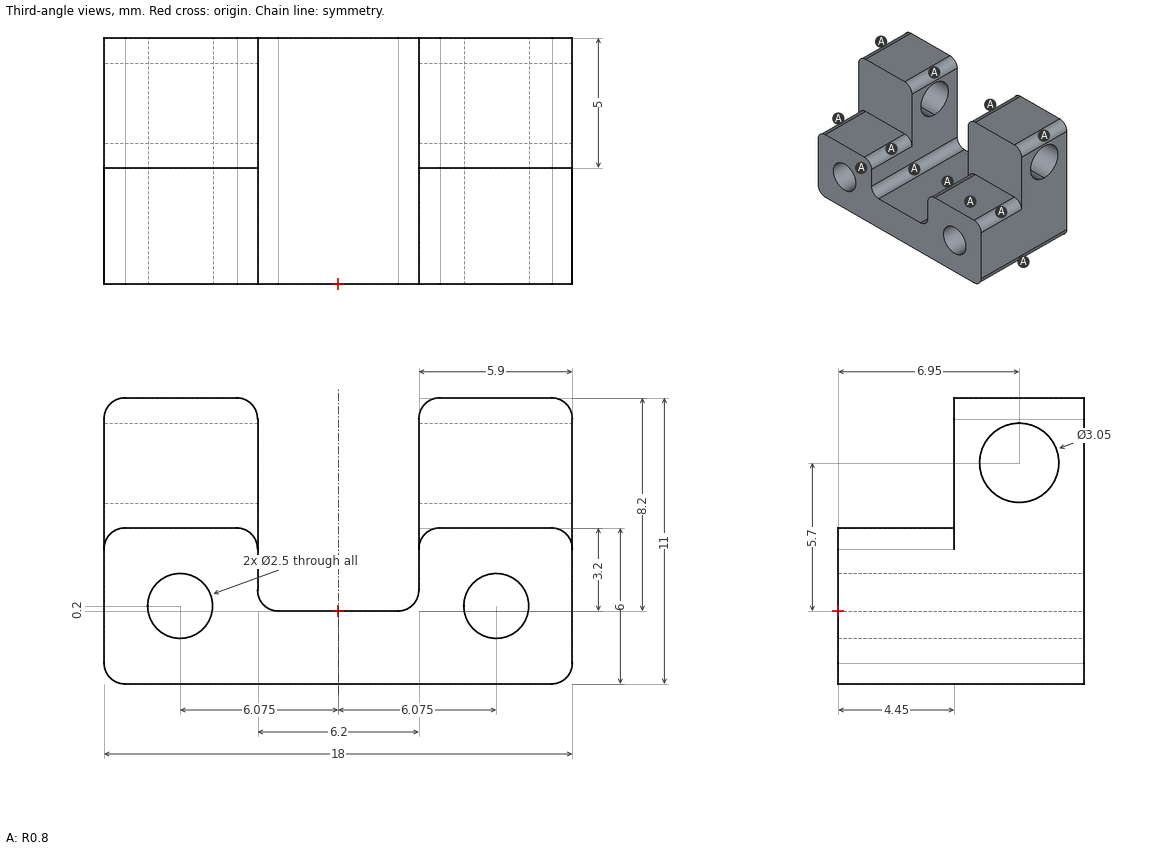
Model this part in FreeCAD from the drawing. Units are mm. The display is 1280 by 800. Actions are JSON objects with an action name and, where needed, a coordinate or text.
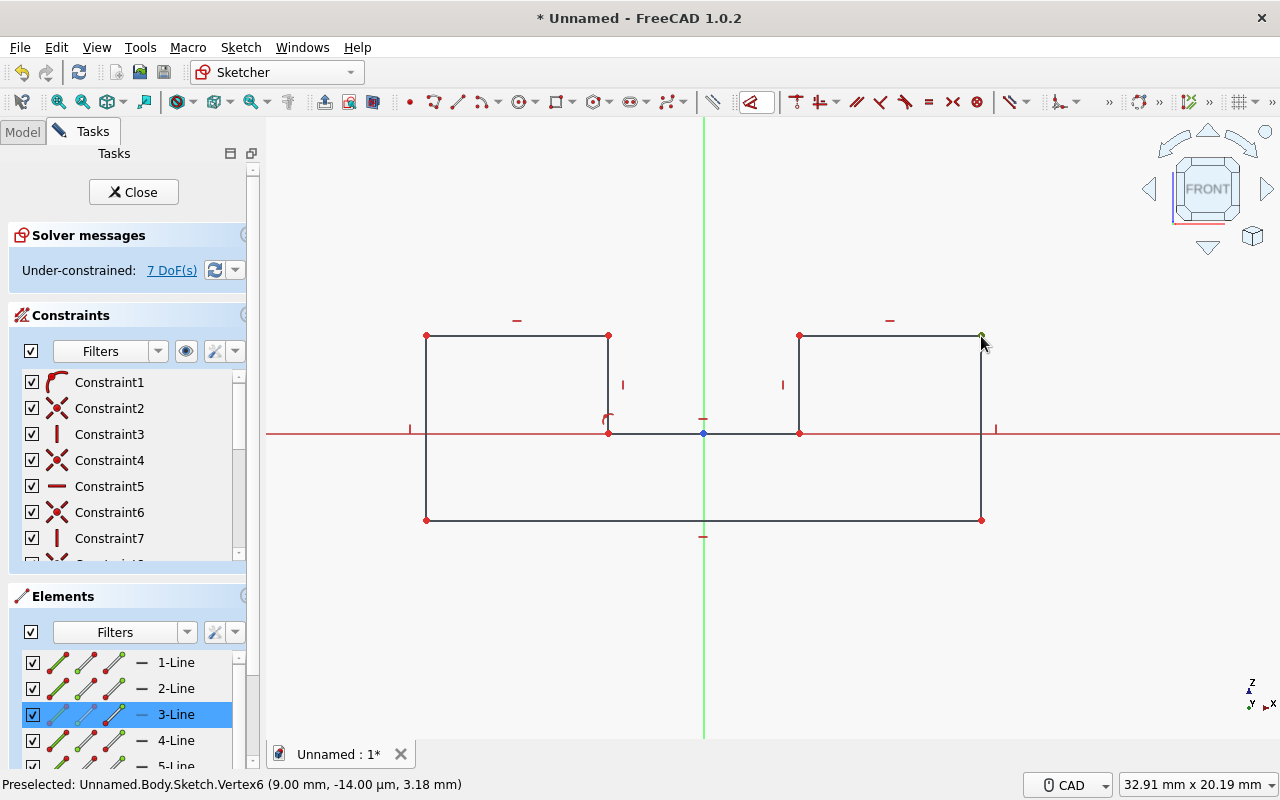
{"action": "left_click", "coordinate": [426, 336]}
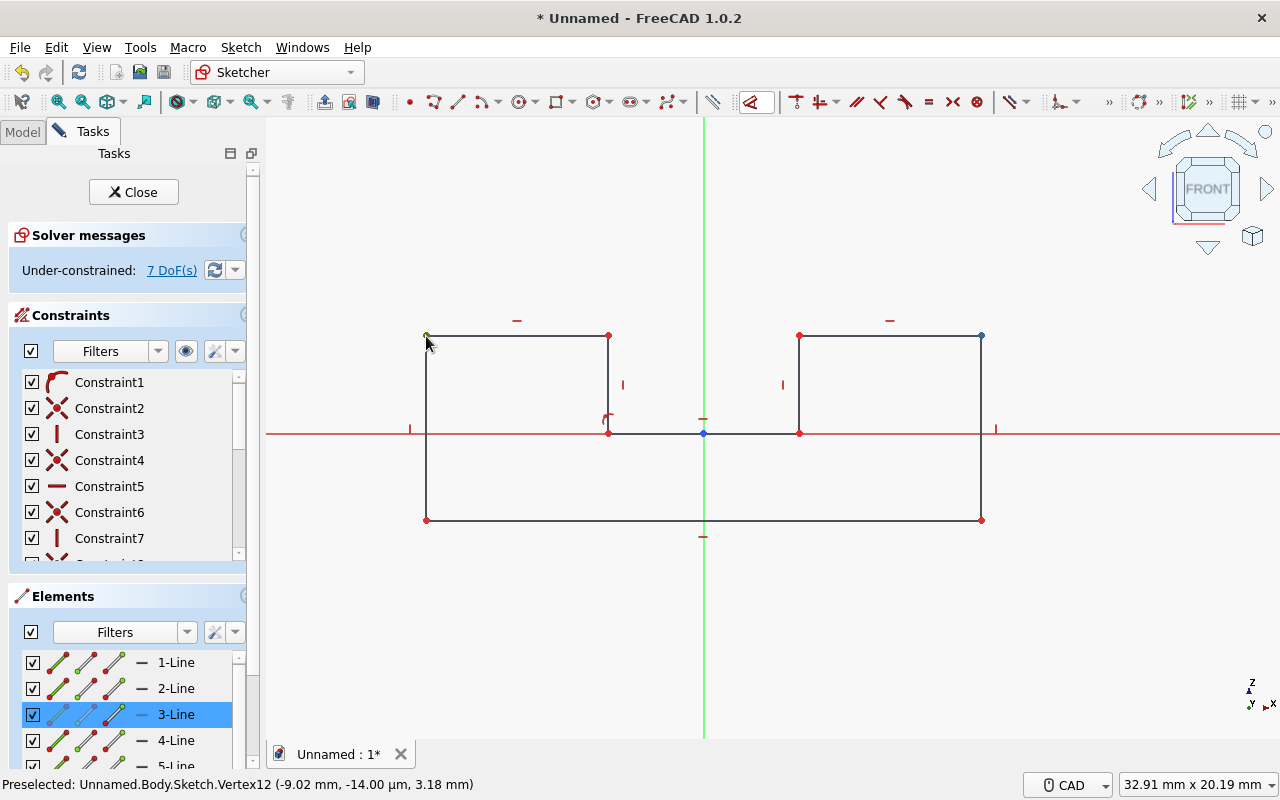
{"action": "left_click", "coordinate": [704, 671]}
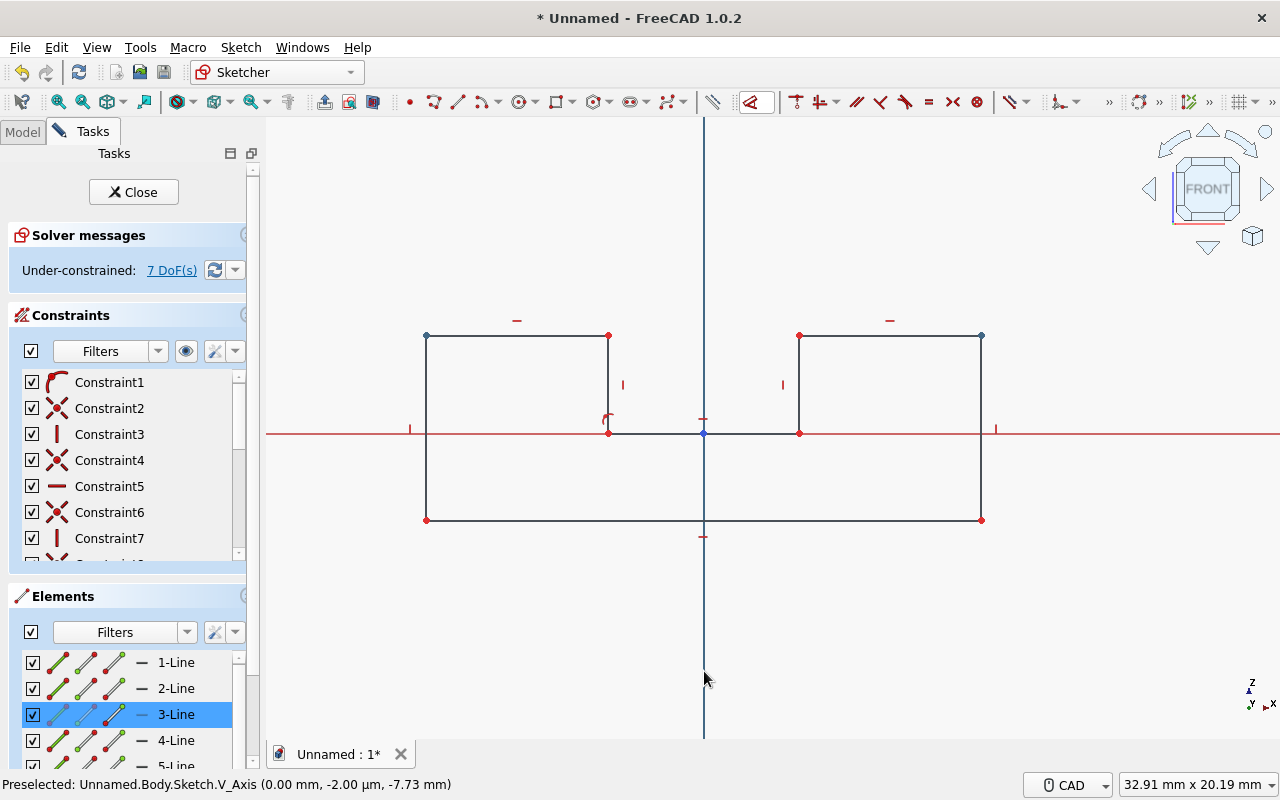
{"action": "left_click", "coordinate": [954, 102]}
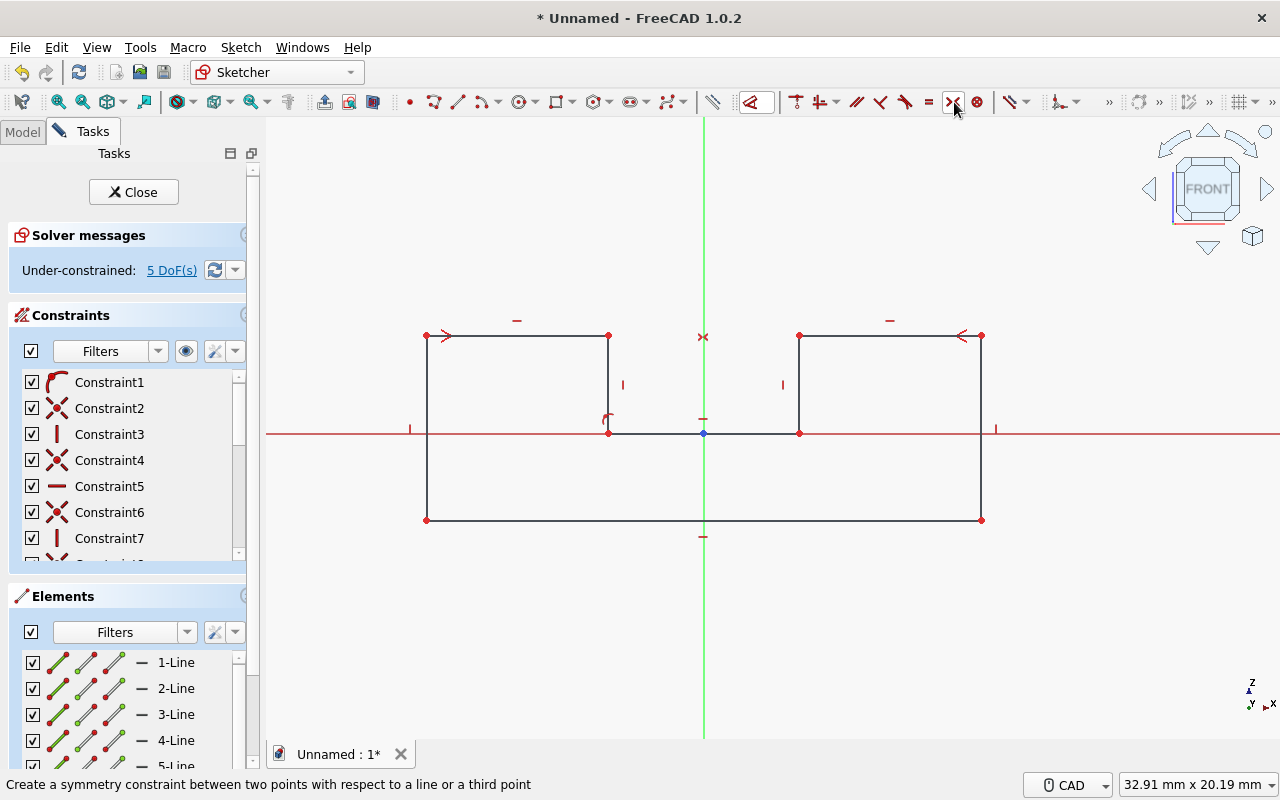
{"action": "left_click", "coordinate": [750, 102]}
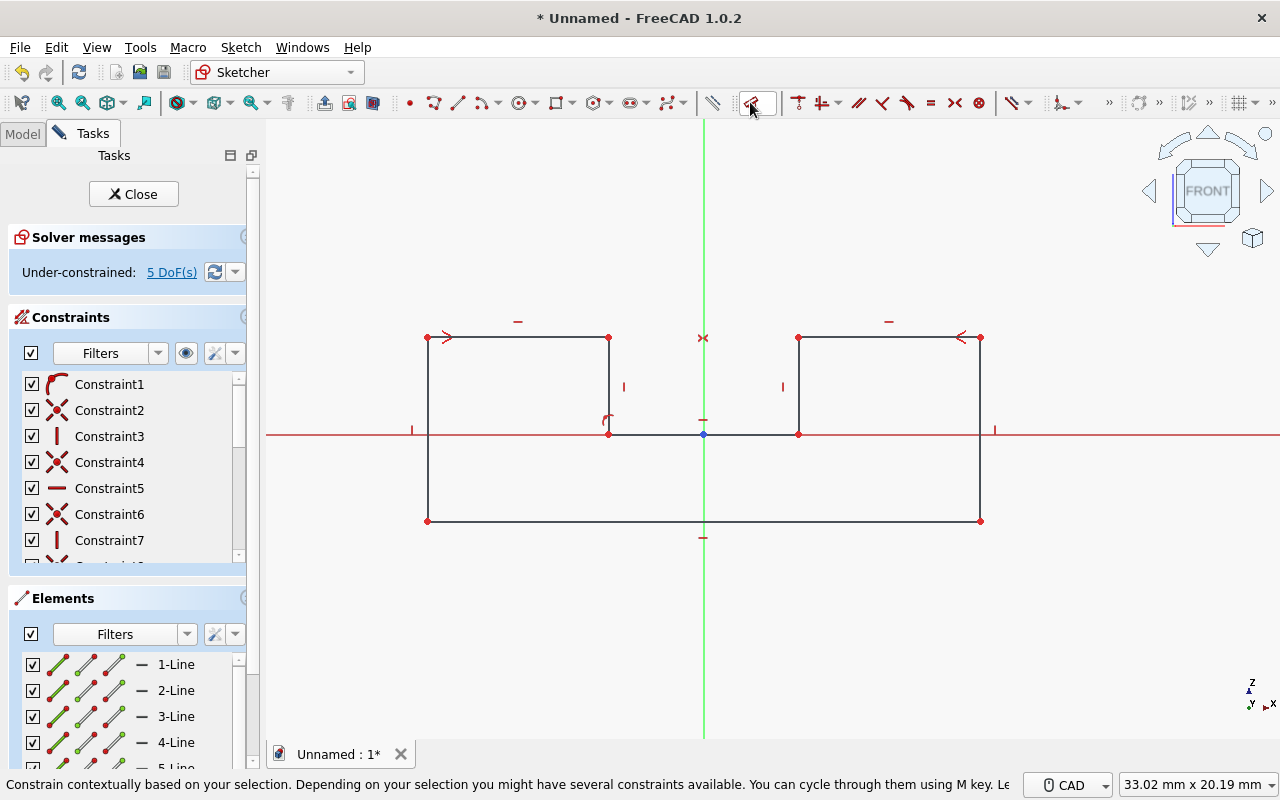
{"action": "left_click", "coordinate": [980, 393]}
{"action": "left_click", "coordinate": [1014, 387]}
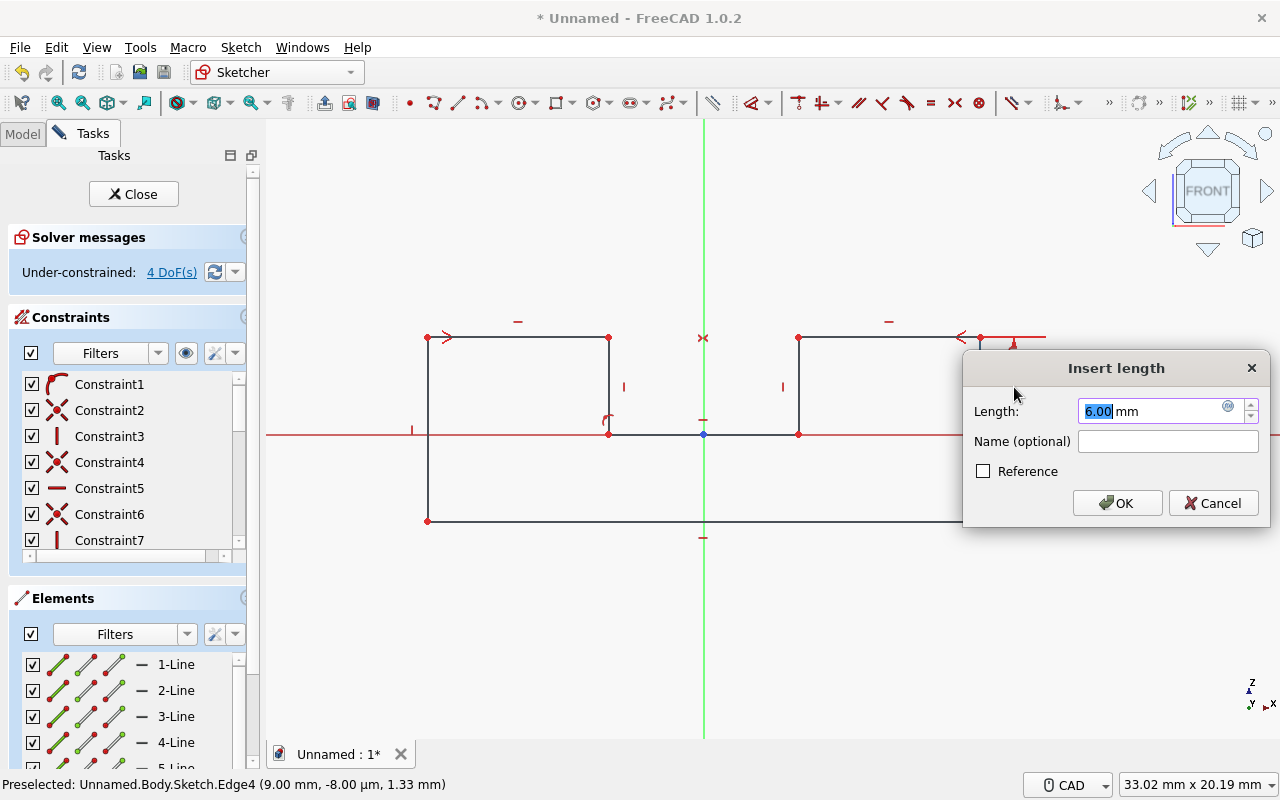
{"action": "type", "text": "6"}
{"action": "key", "text": "Return"}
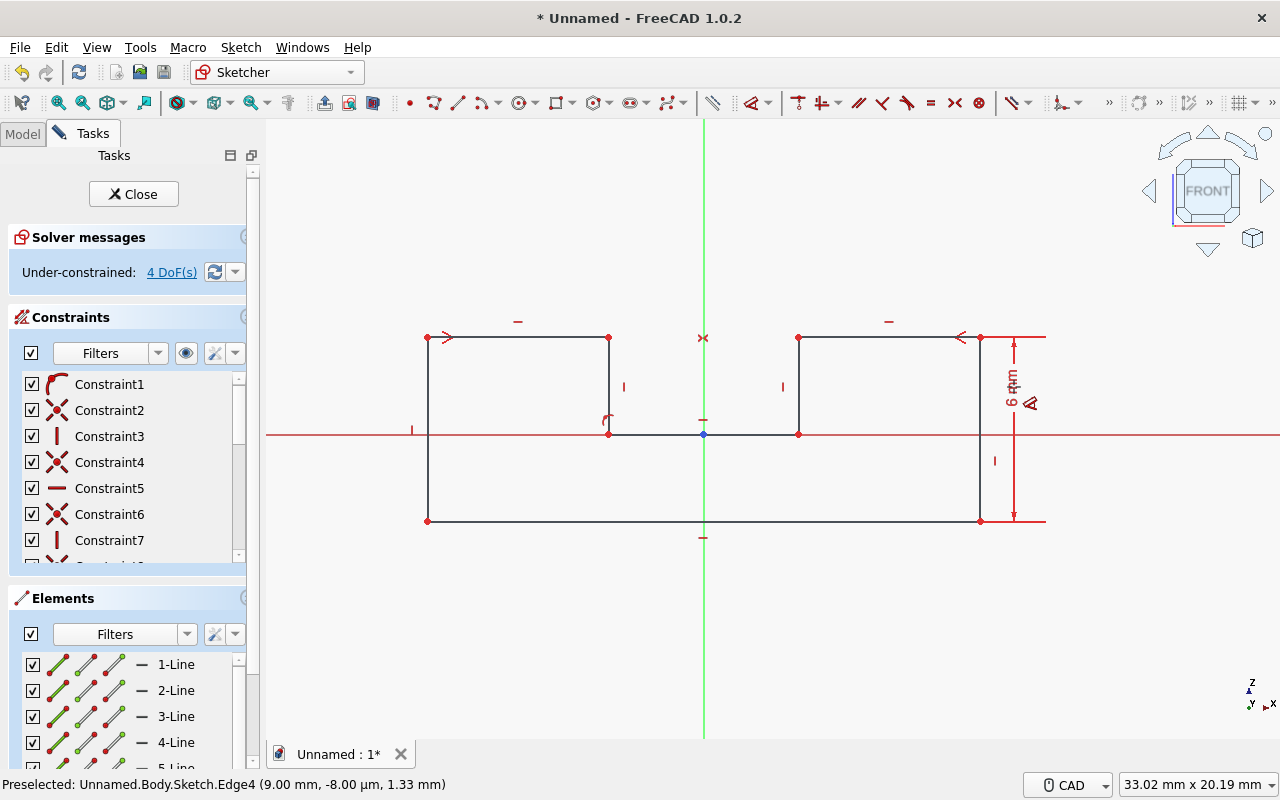
{"action": "left_click", "coordinate": [815, 522]}
{"action": "left_click", "coordinate": [577, 556]}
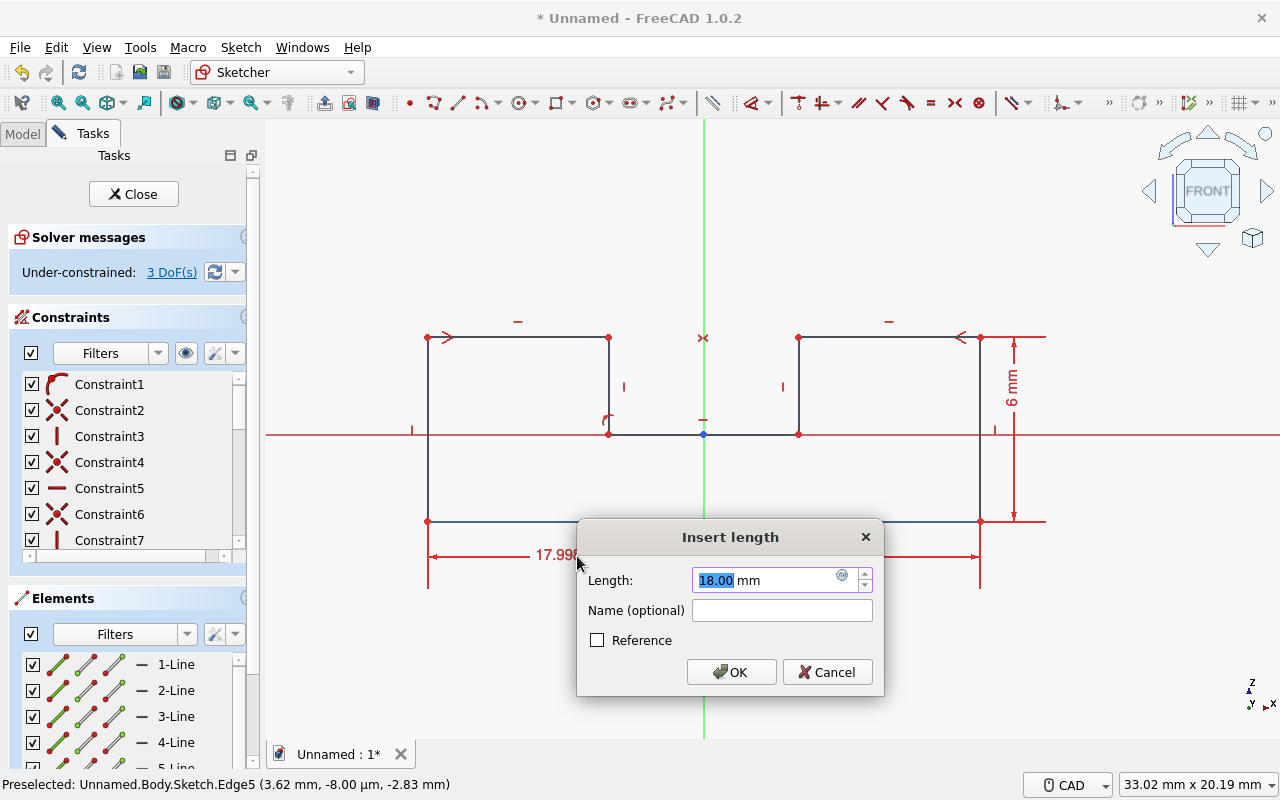
{"action": "type", "text": "18"}
{"action": "key", "text": "Return"}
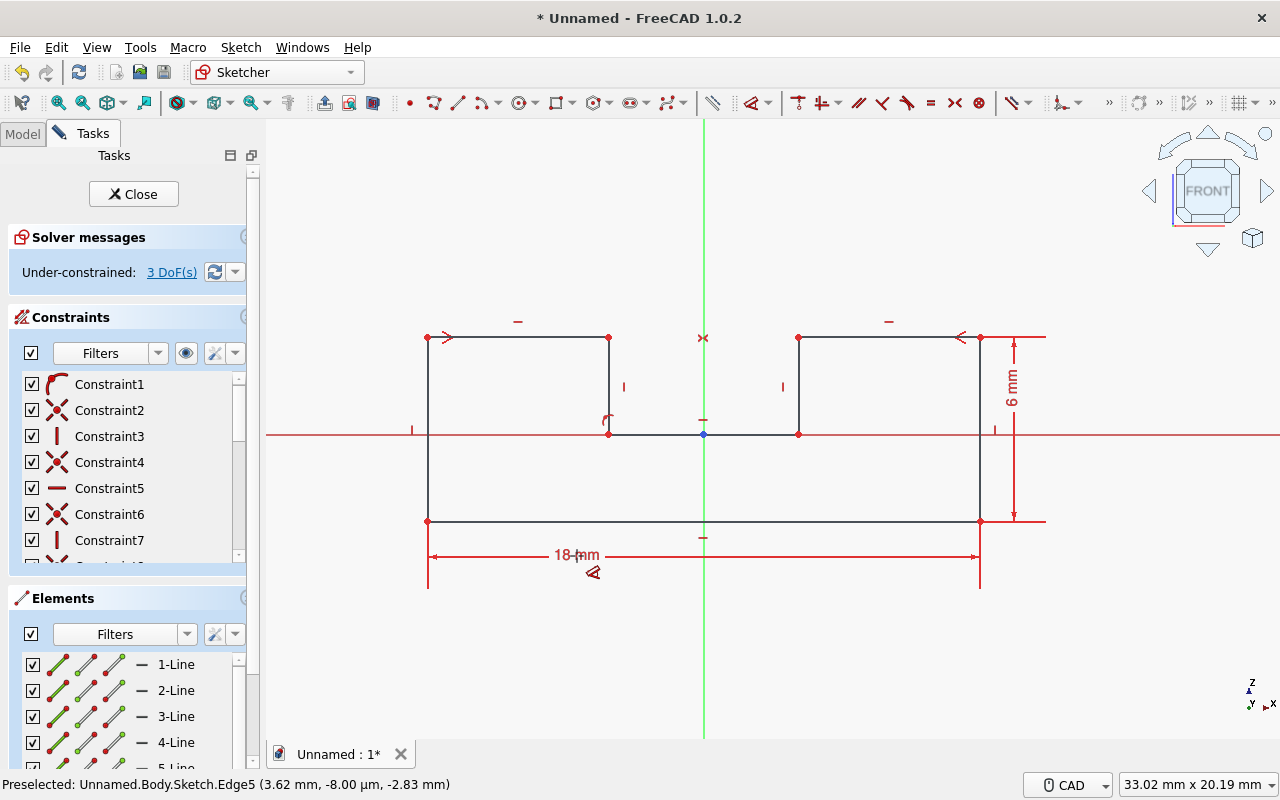
{"action": "left_click", "coordinate": [666, 435]}
{"action": "left_click", "coordinate": [660, 469]}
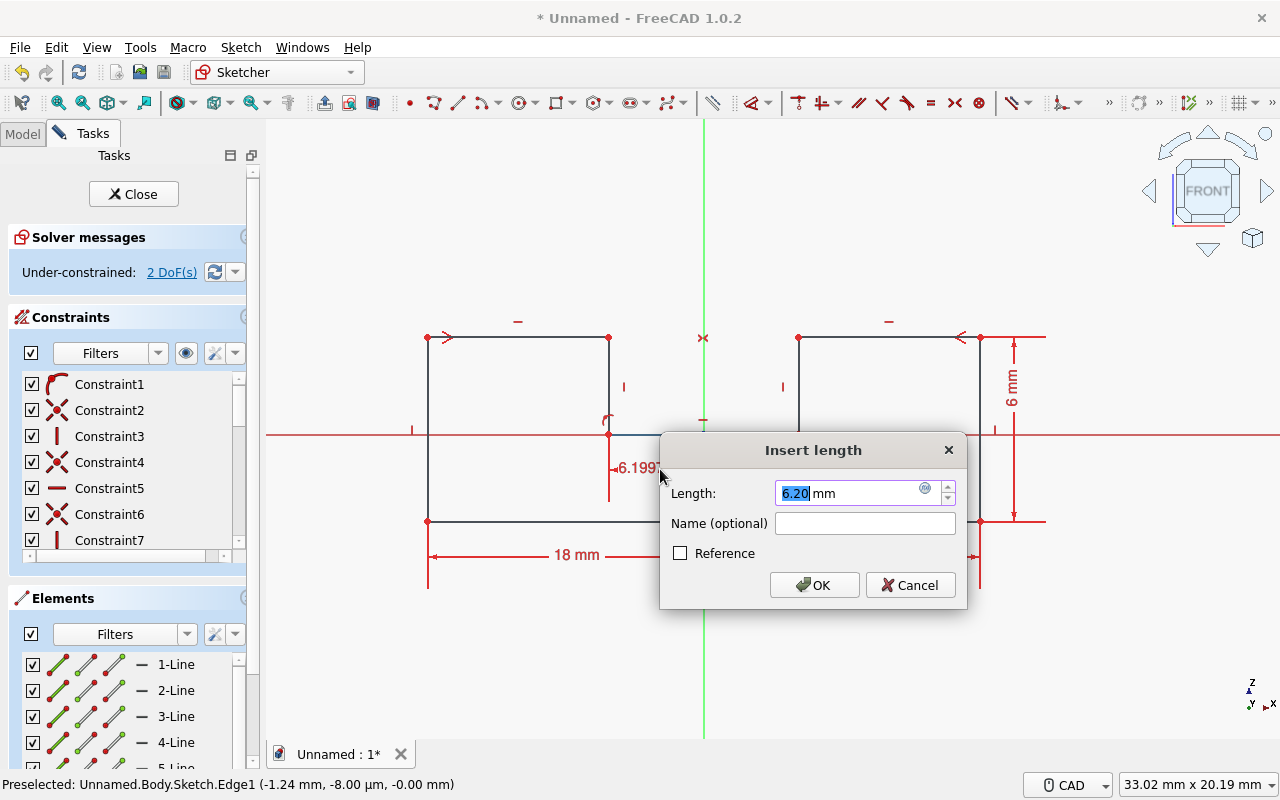
{"action": "type", "text": "6.2"}
{"action": "key", "text": "Return"}